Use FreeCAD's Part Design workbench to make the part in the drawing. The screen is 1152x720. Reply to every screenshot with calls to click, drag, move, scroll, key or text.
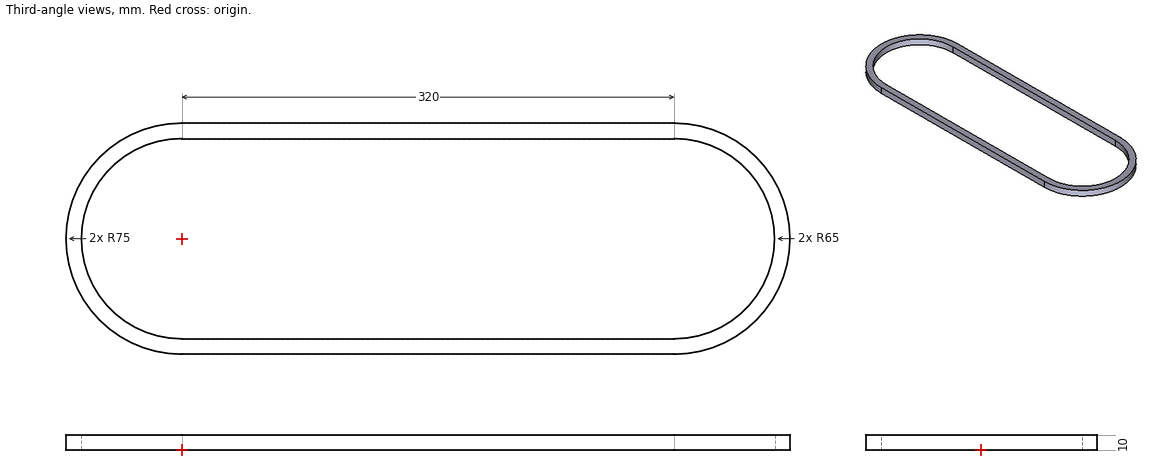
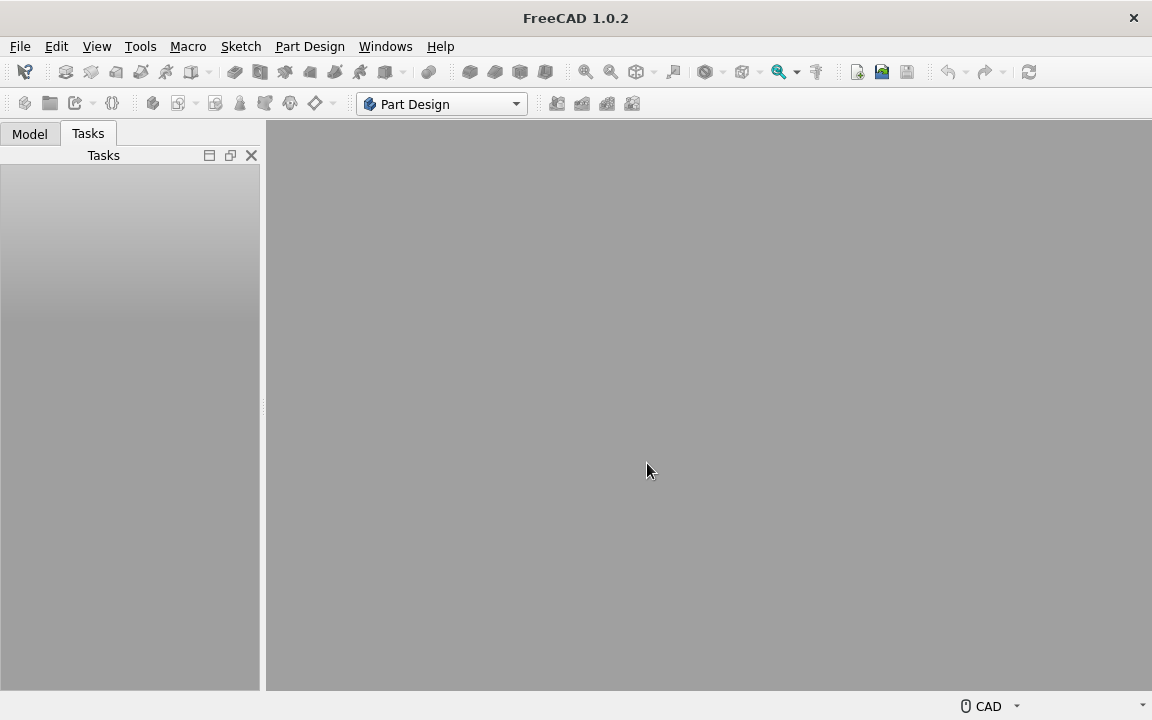
click(857, 72)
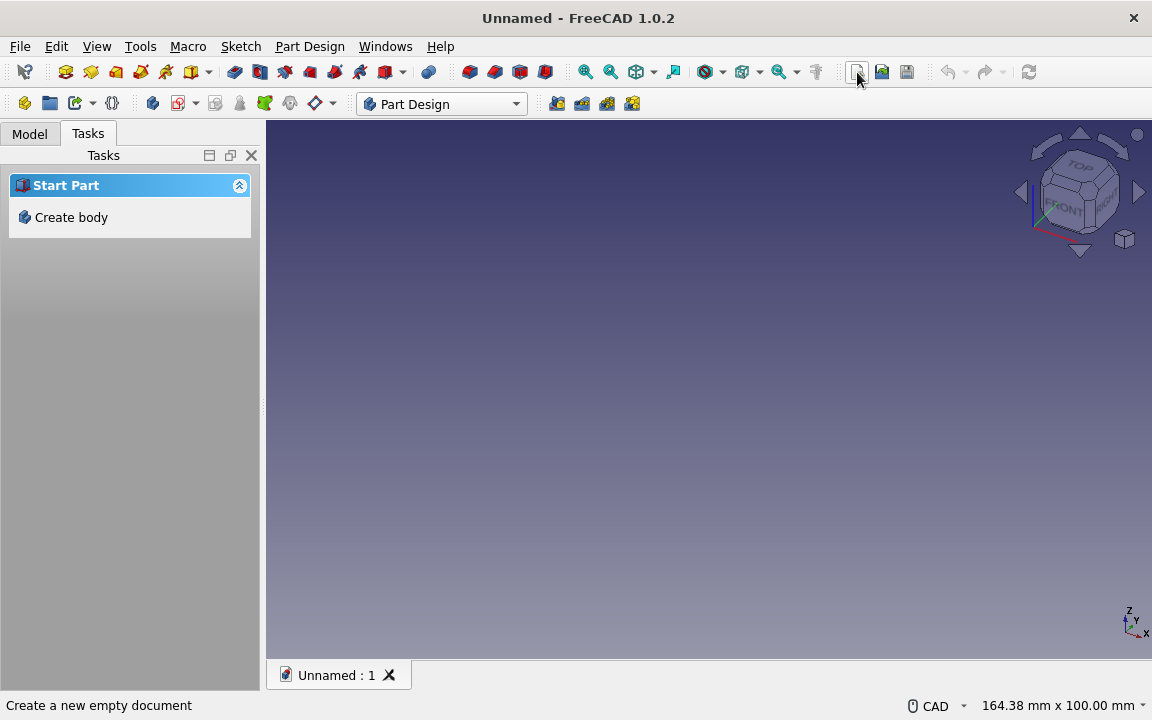
click(178, 104)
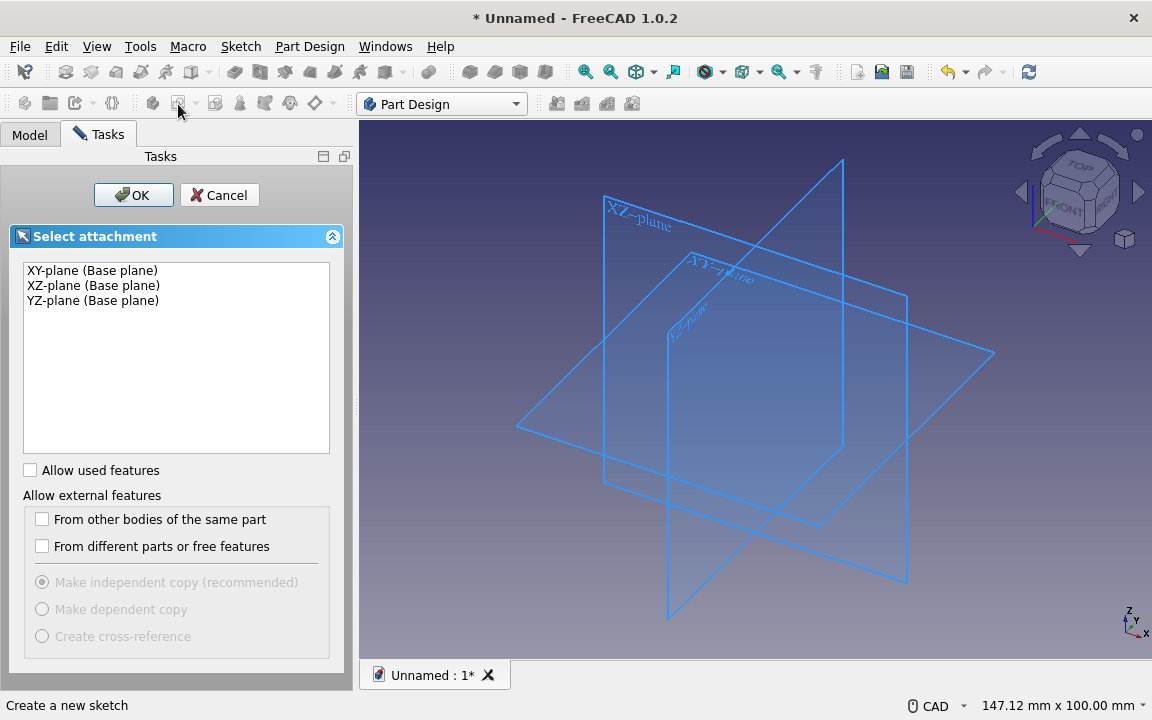
click(84, 270)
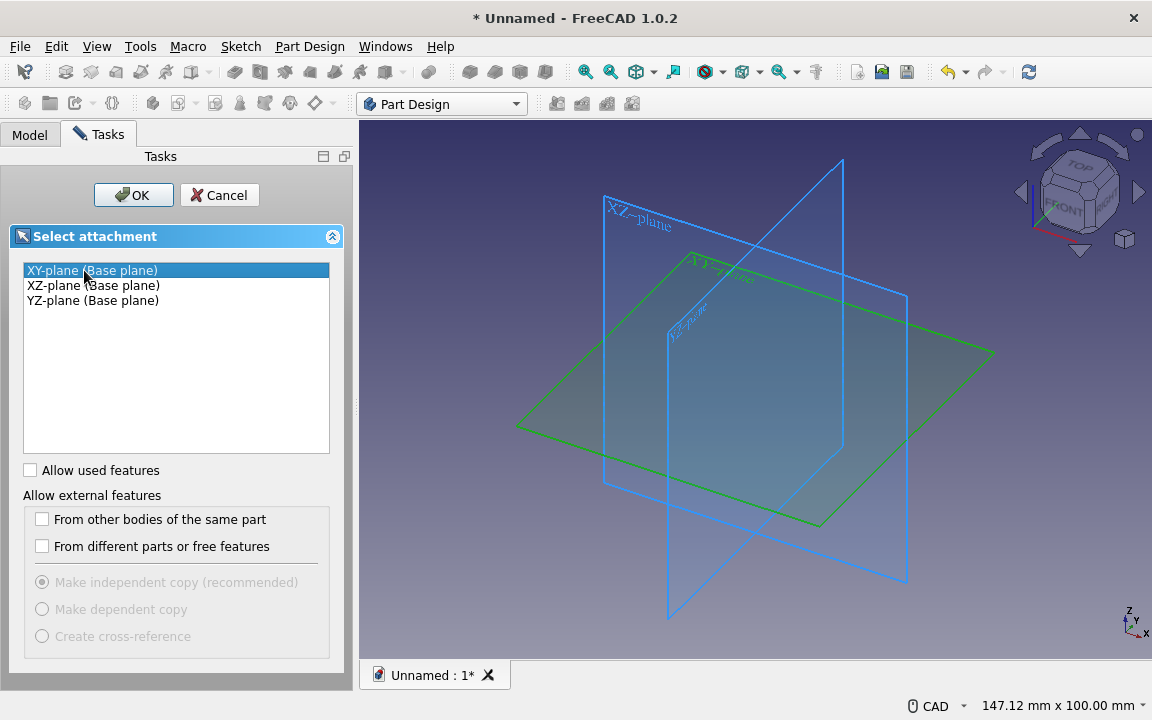
click(134, 195)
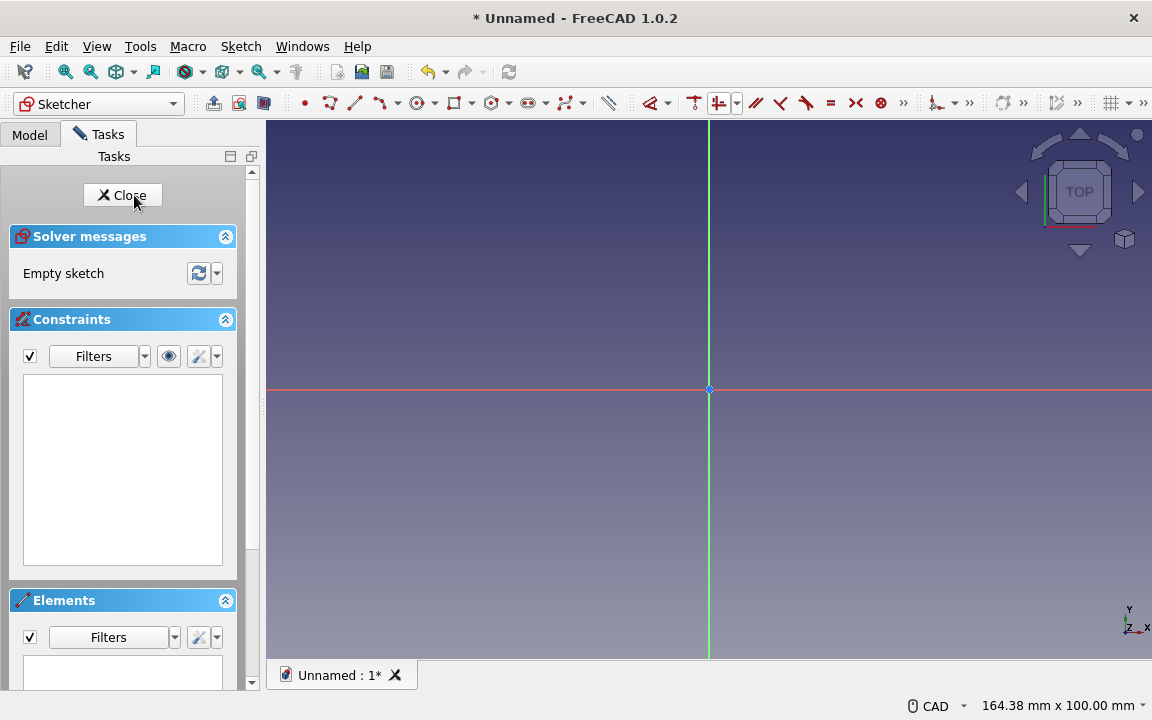
scroll(405, 389, down, 8)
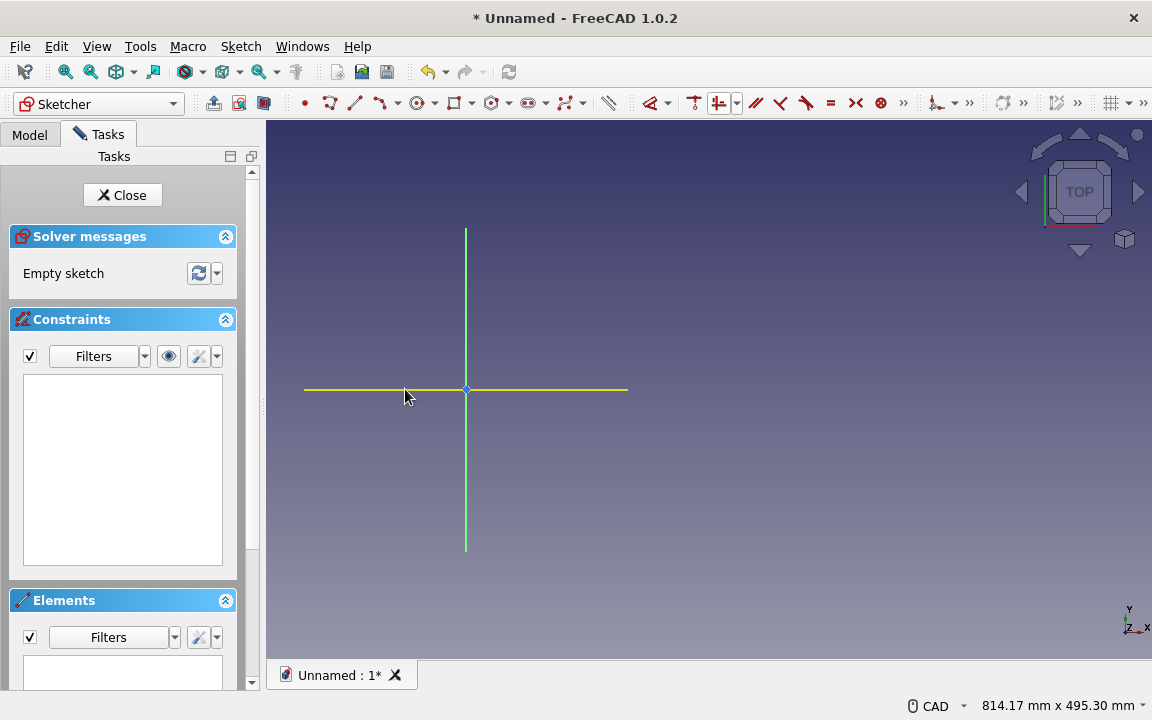
click(528, 104)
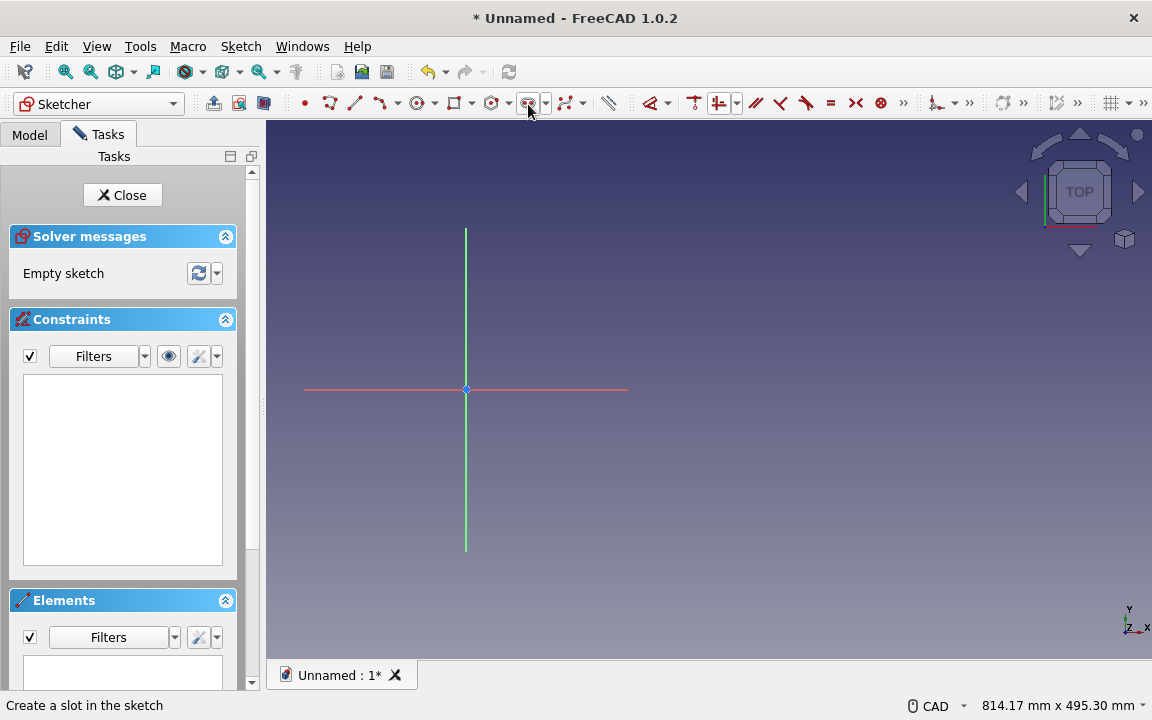
click(467, 390)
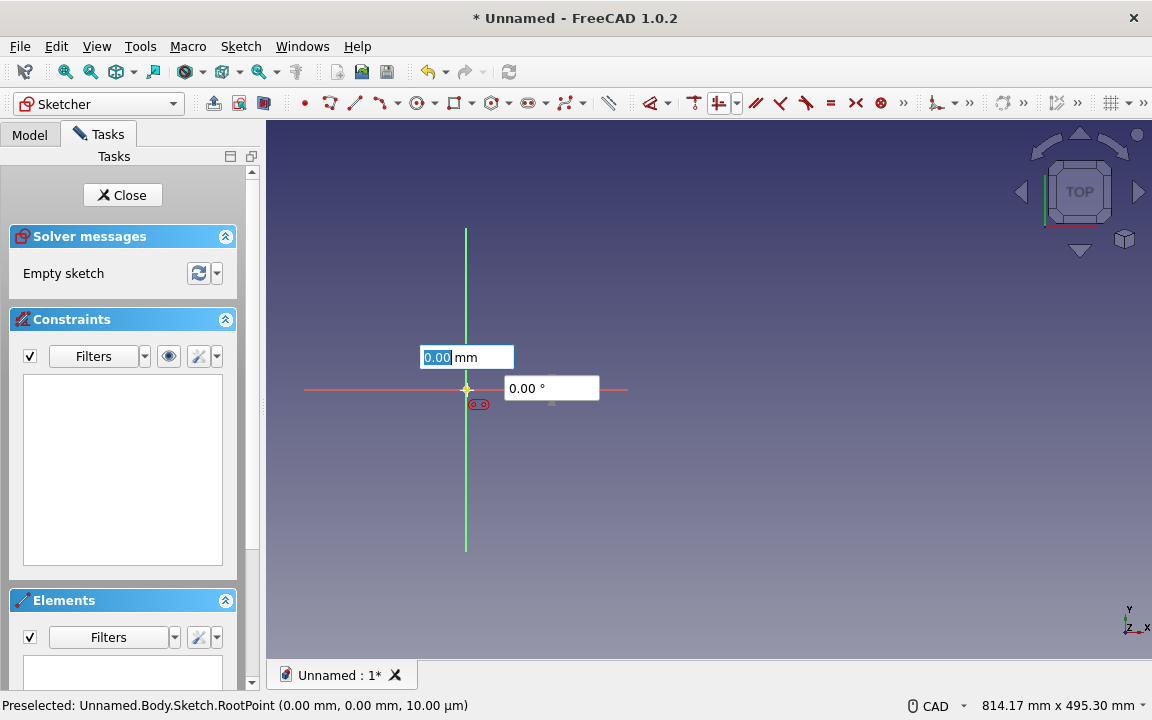
click(815, 380)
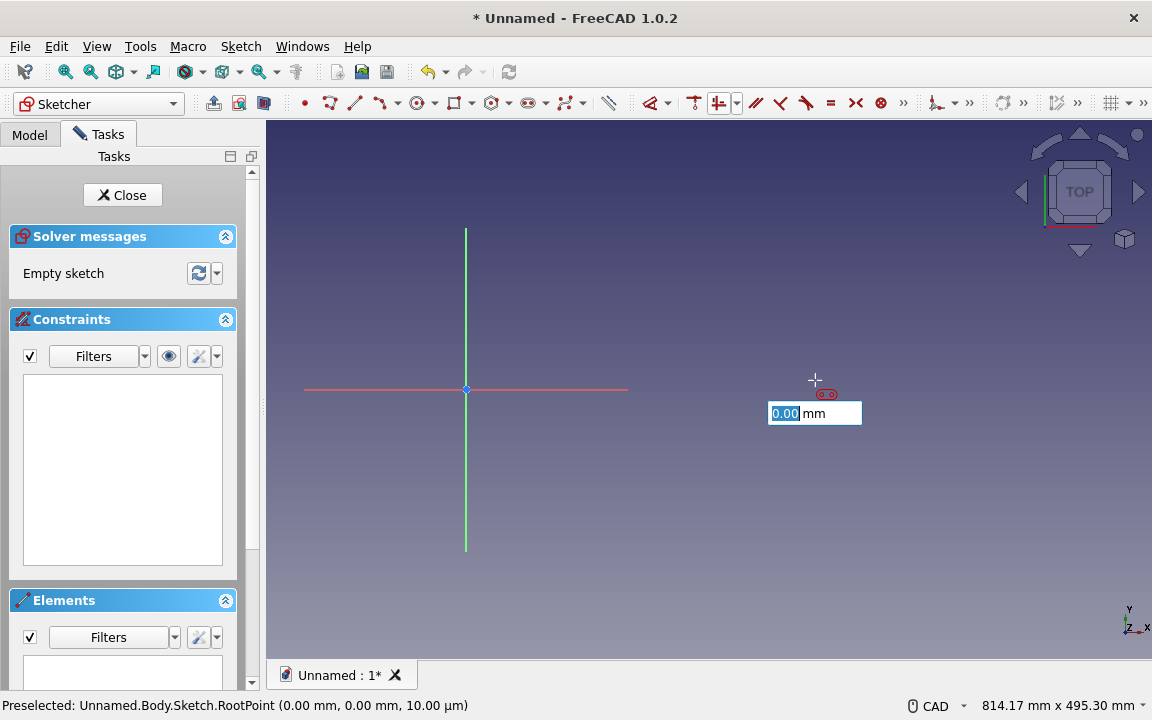
click(641, 308)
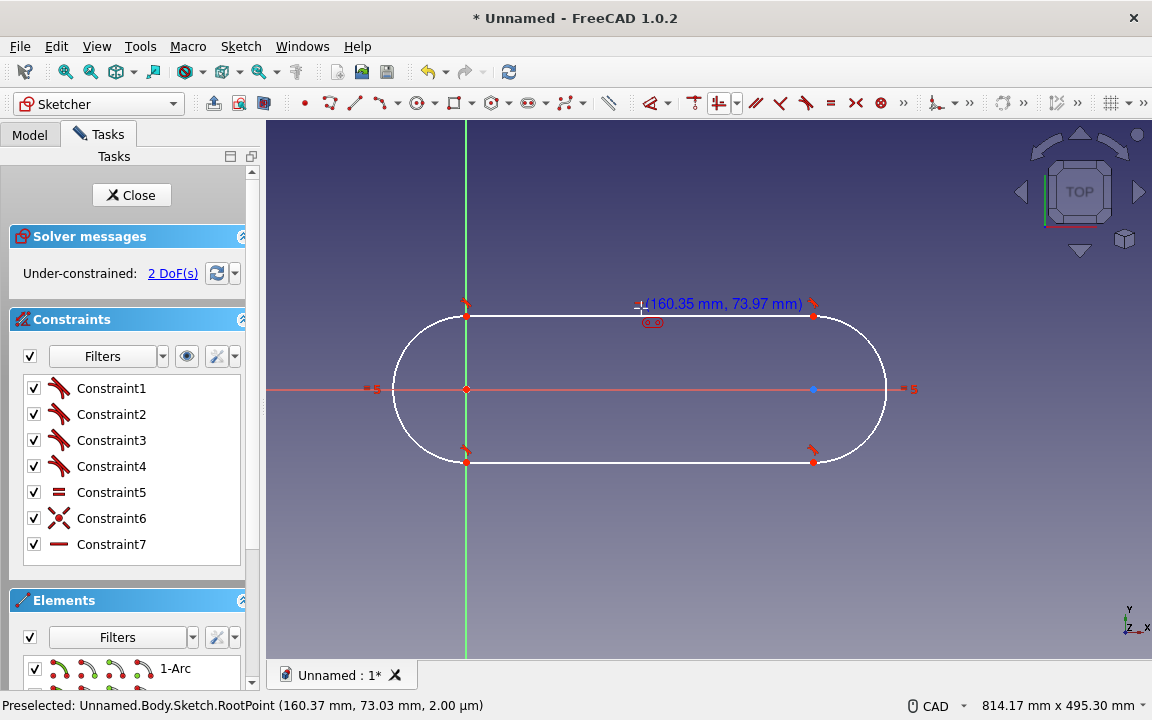
click(467, 390)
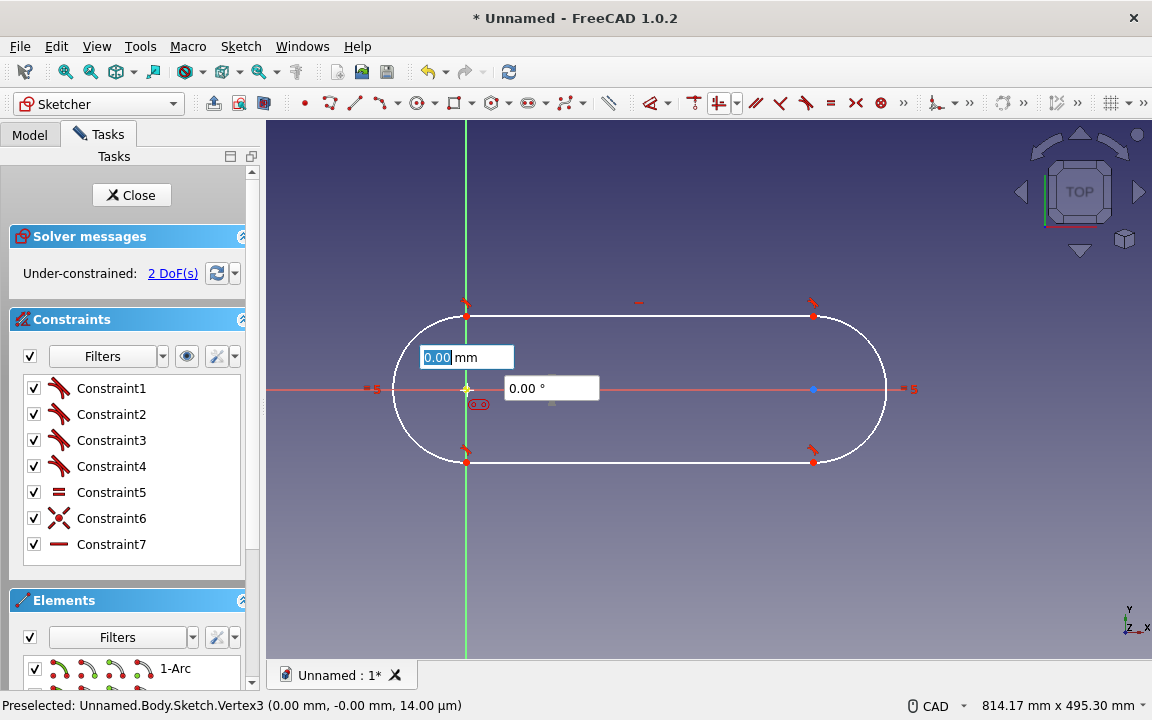
click(815, 380)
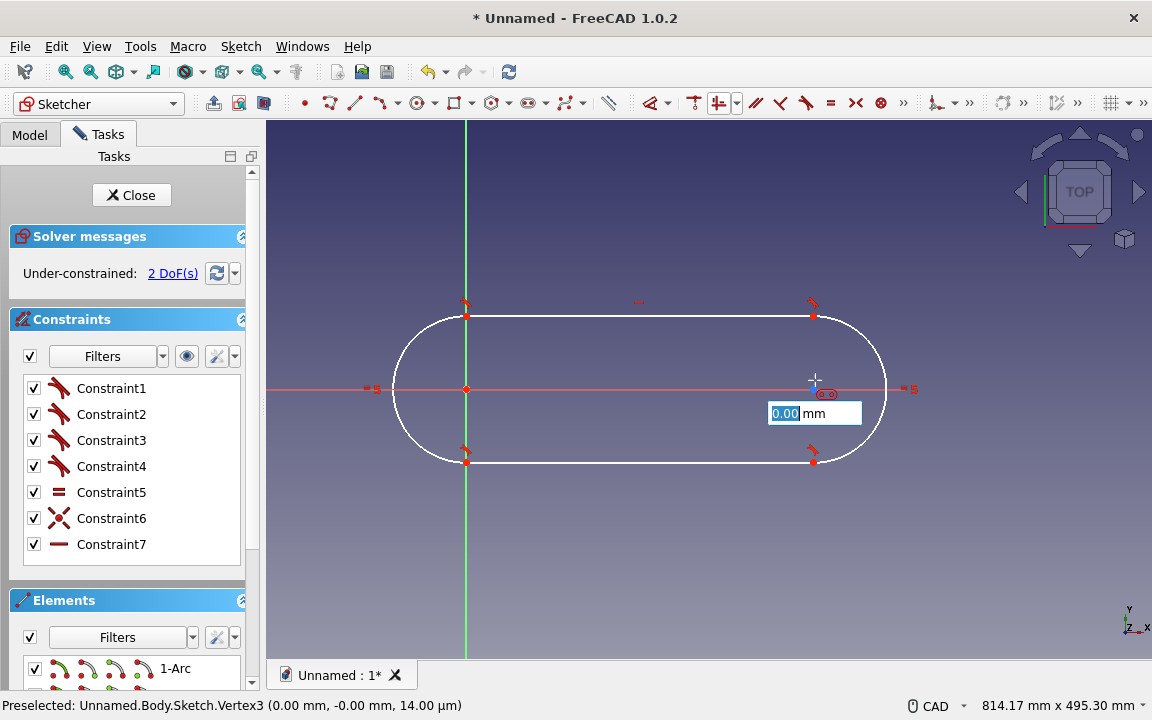
scroll(641, 319, up, 2)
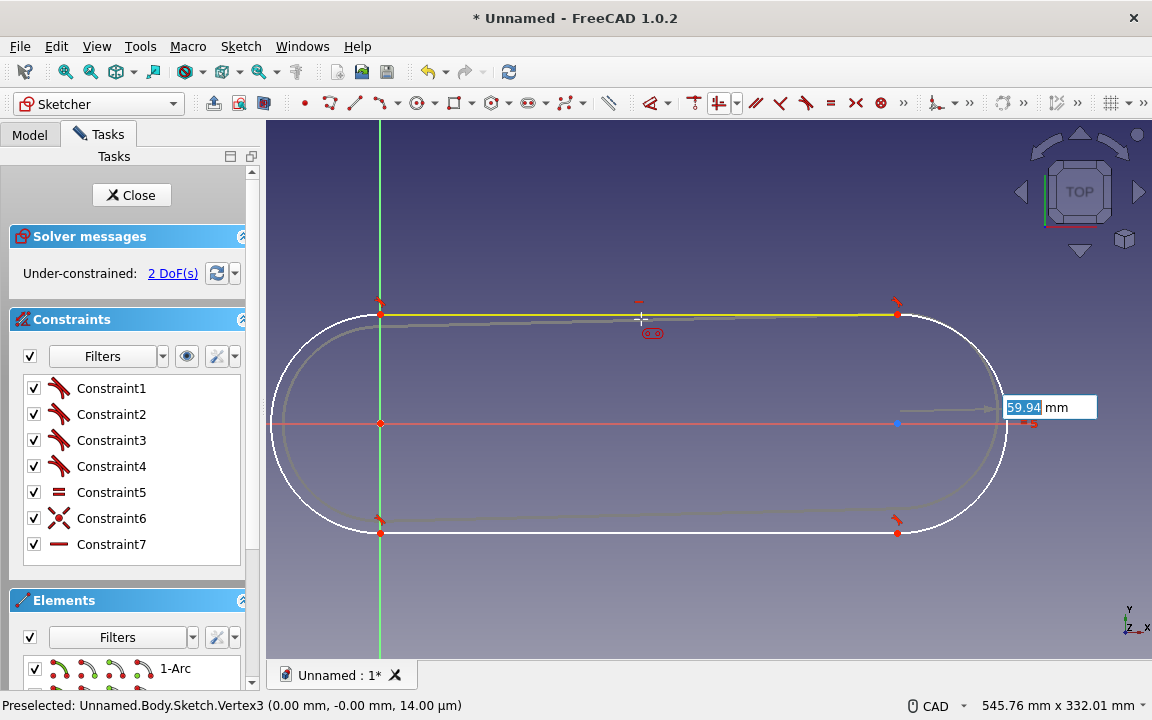
click(640, 318)
key(Escape)